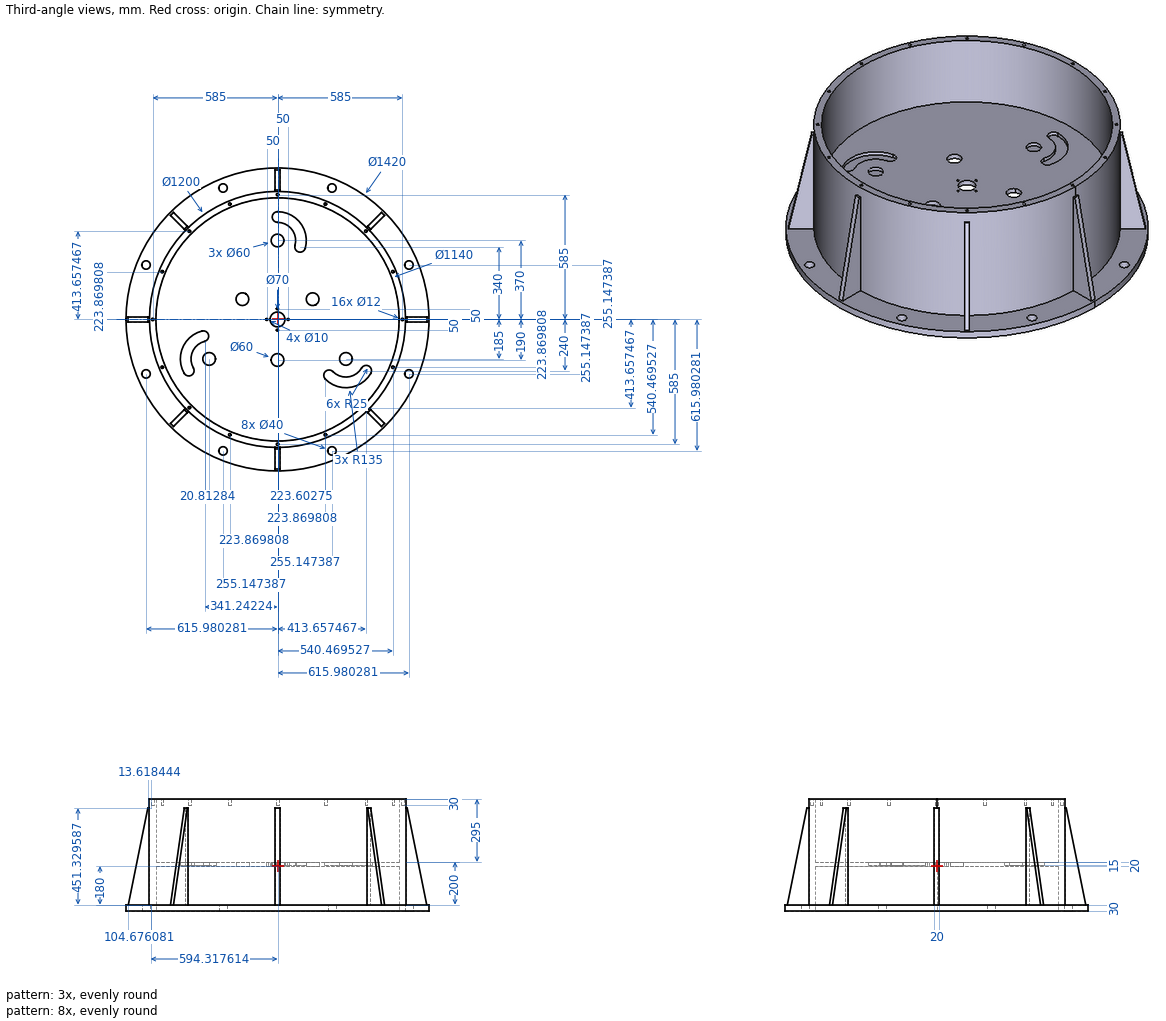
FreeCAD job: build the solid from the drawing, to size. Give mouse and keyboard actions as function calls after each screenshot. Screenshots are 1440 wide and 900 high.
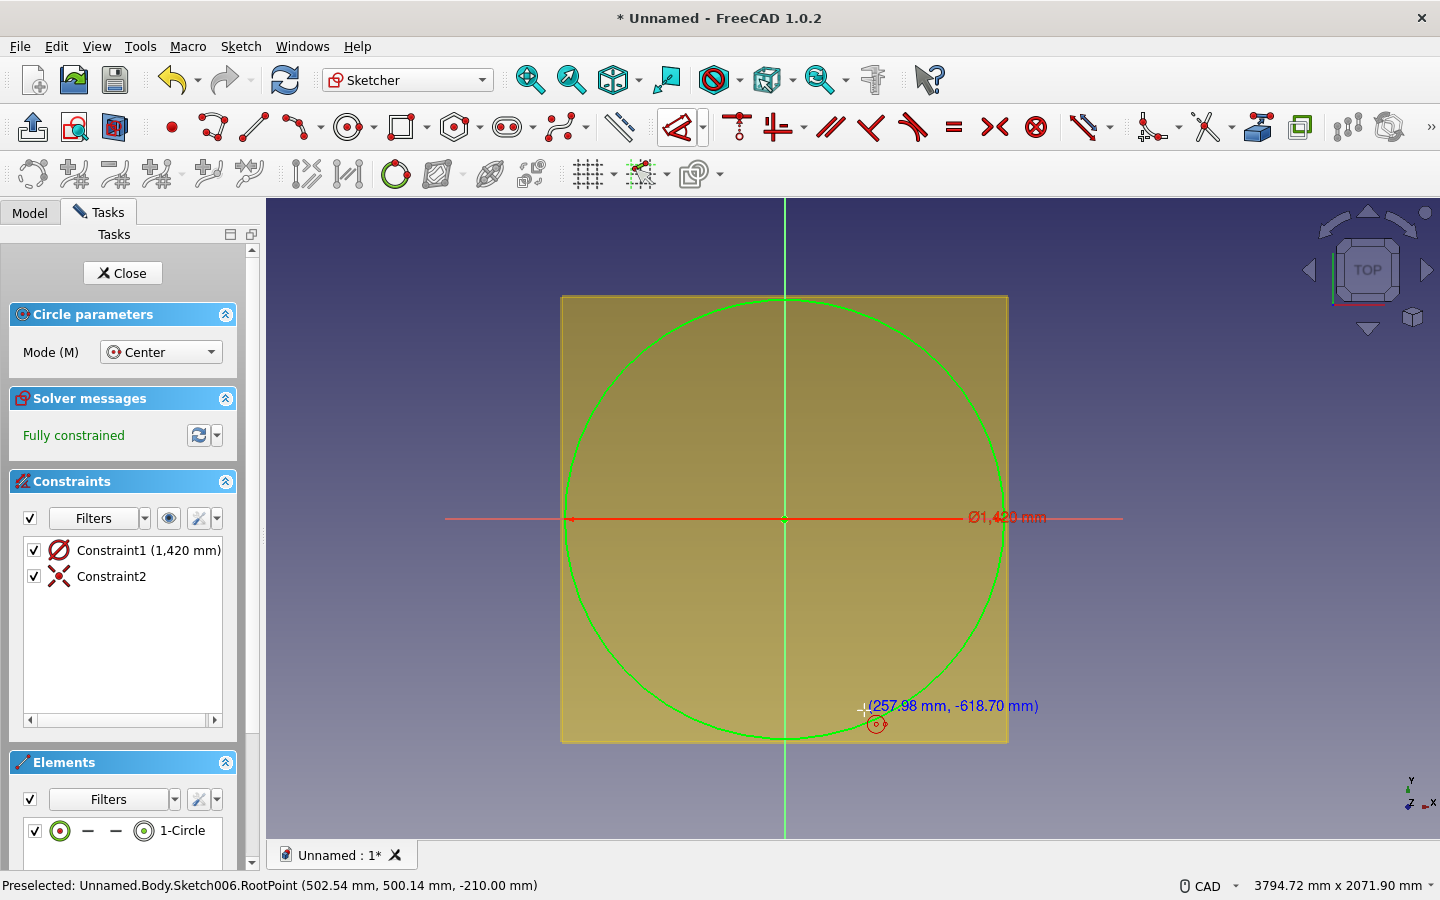
click(864, 710)
move(868, 706)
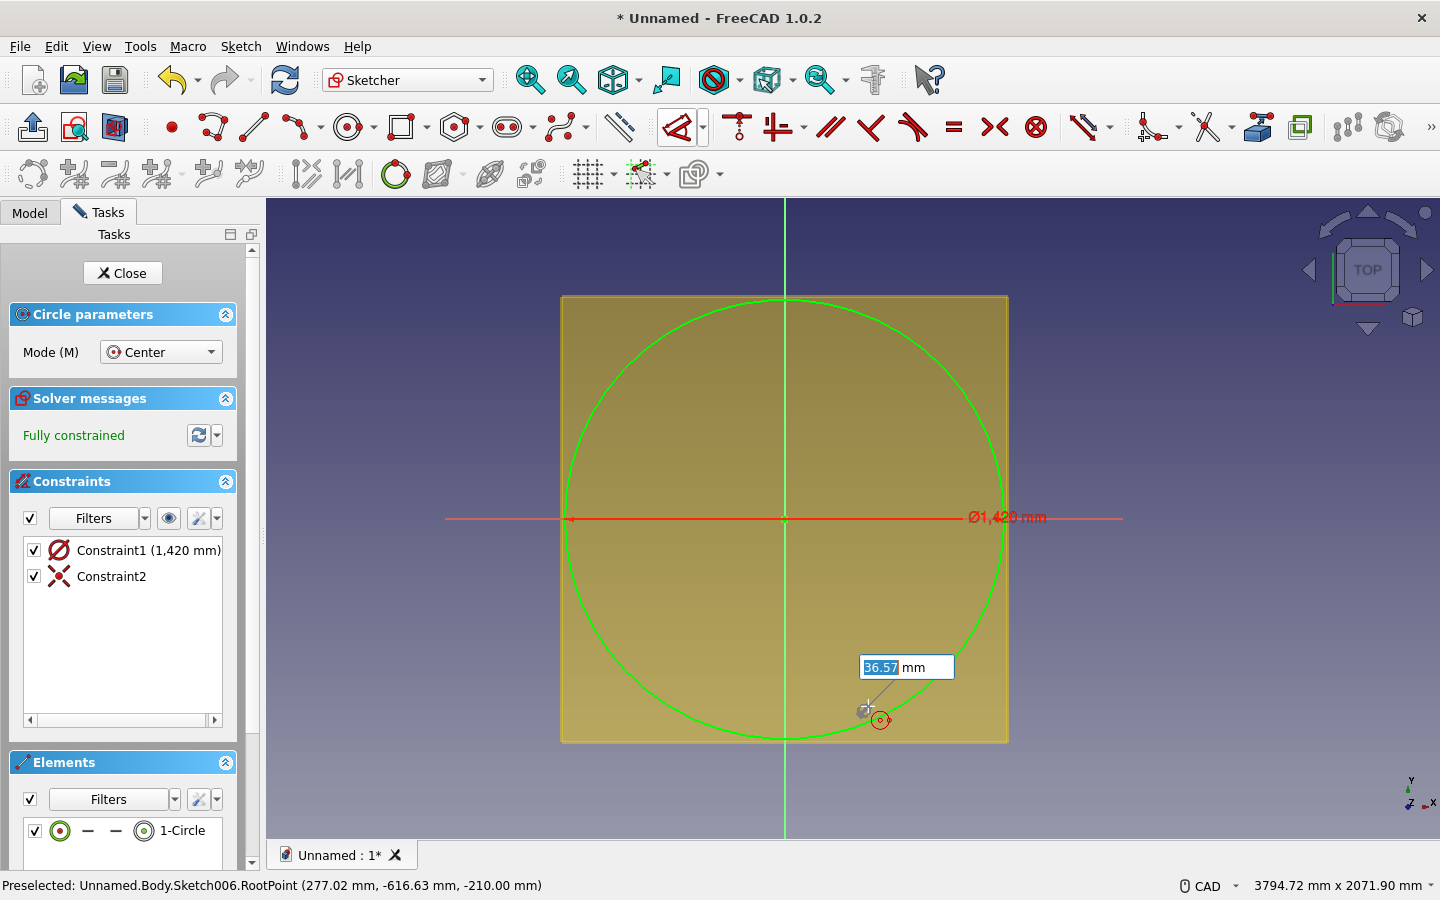
text(40)
key(Return)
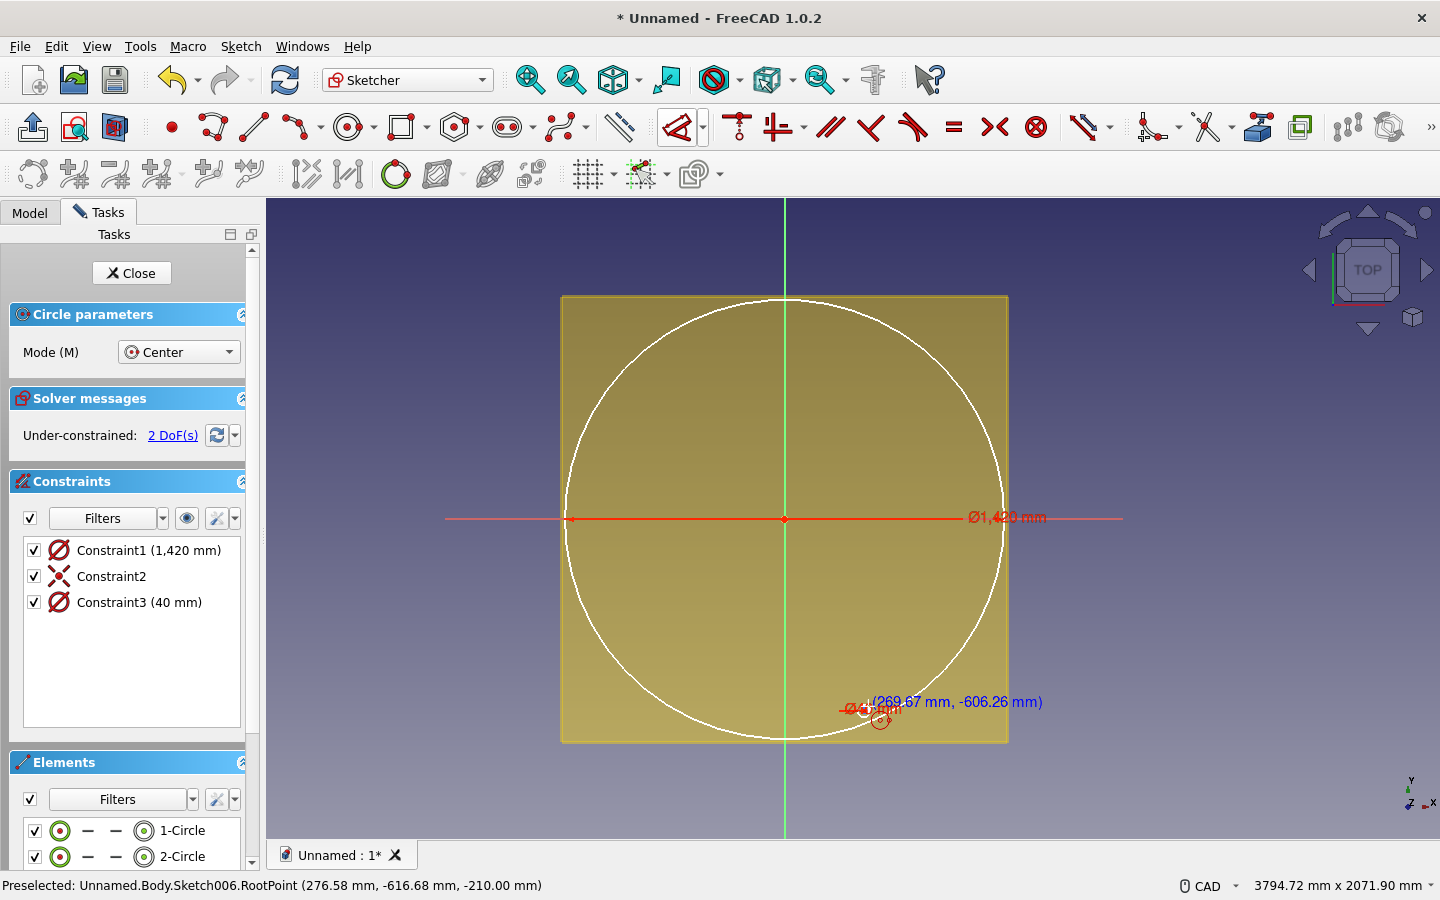
scroll(975, 598, up, 7)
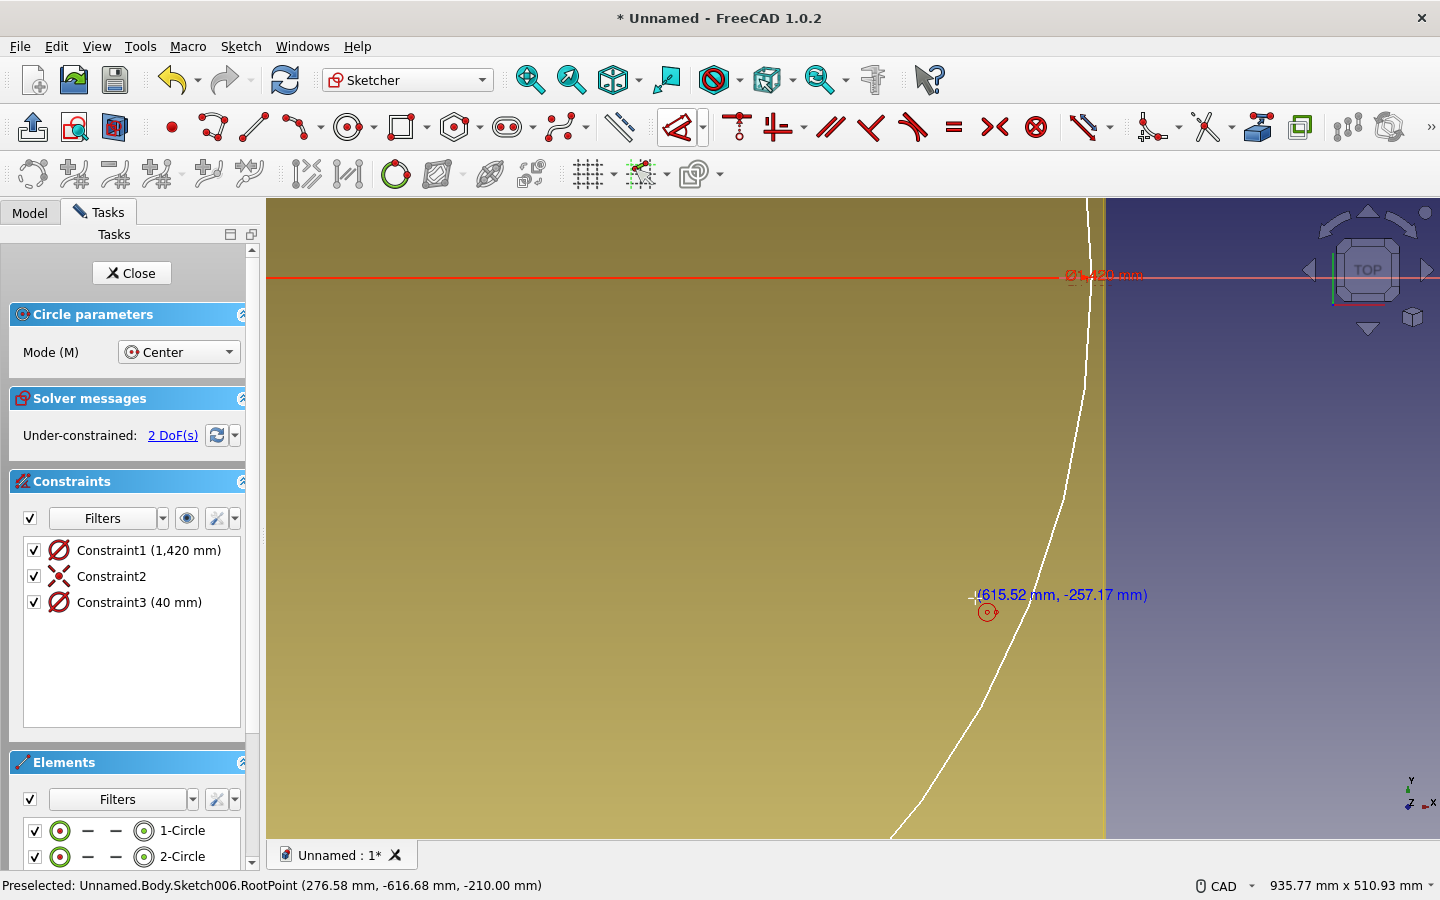
scroll(976, 597, down, 7)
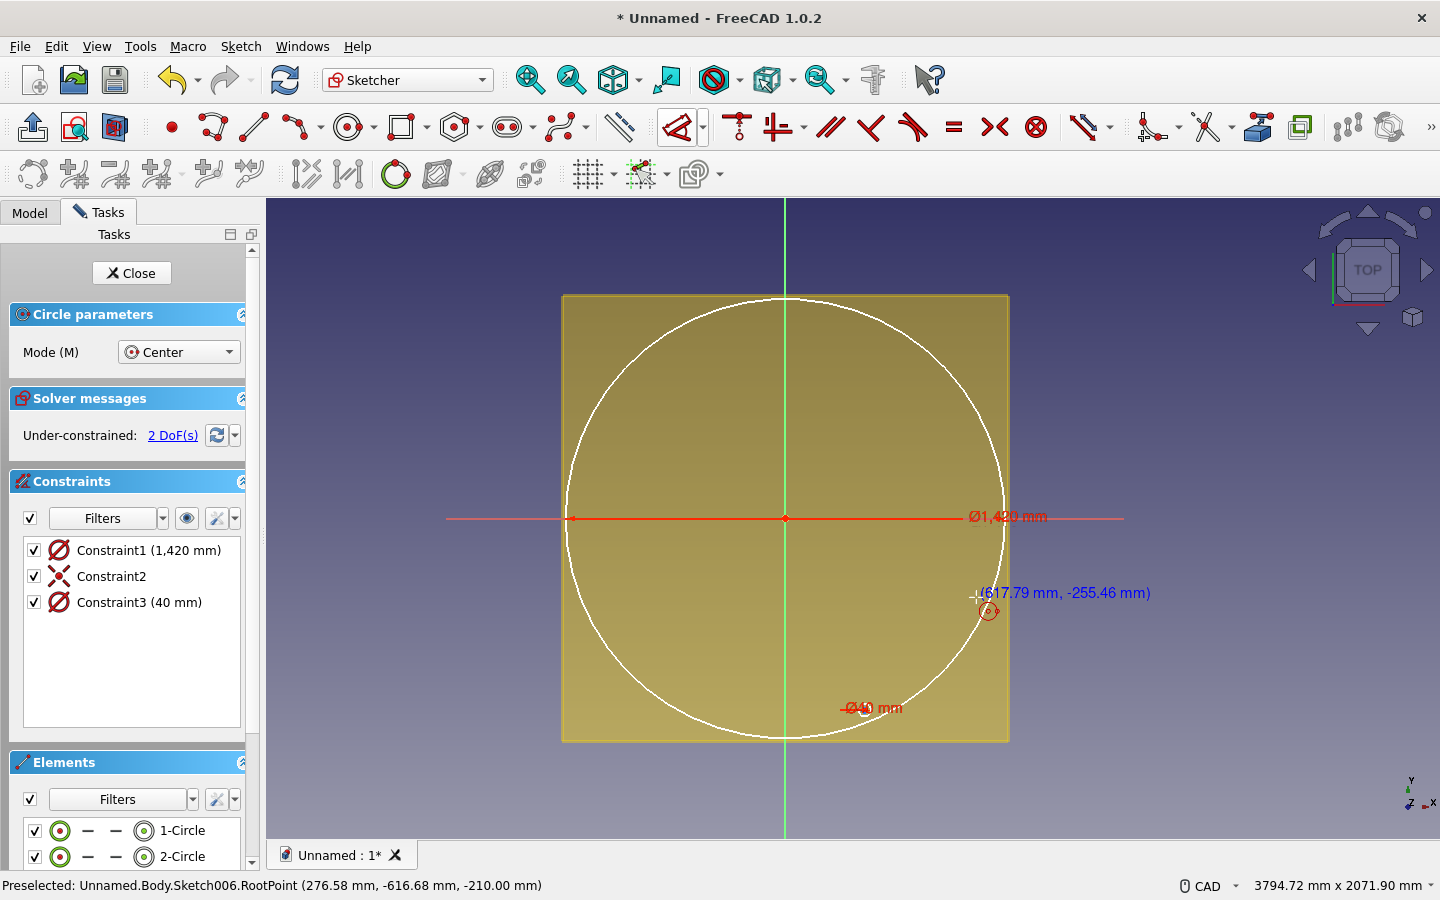
click(976, 598)
move(972, 593)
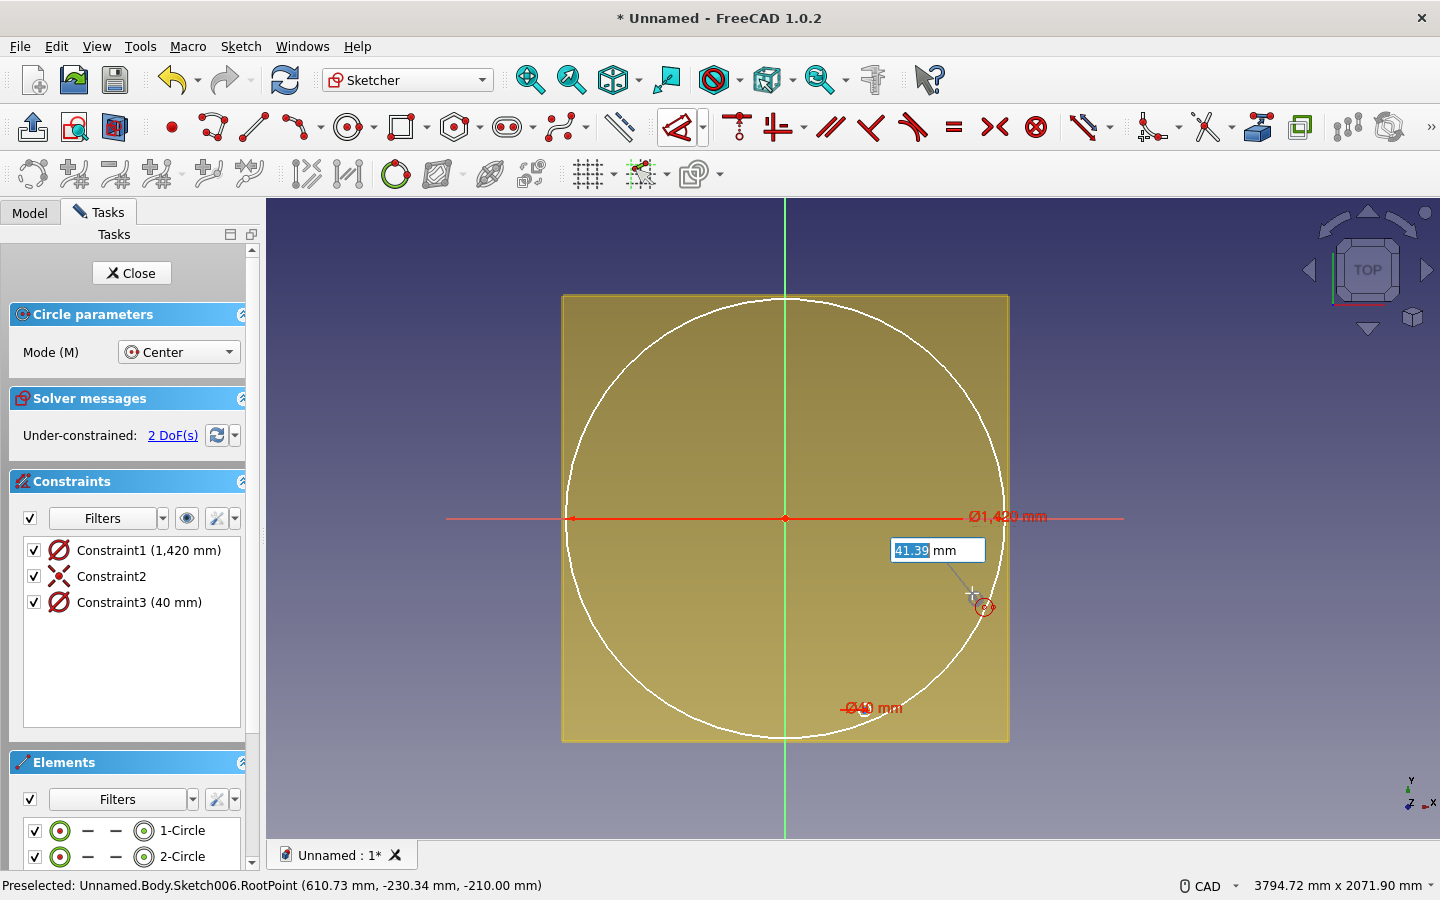
text(40)
key(Return)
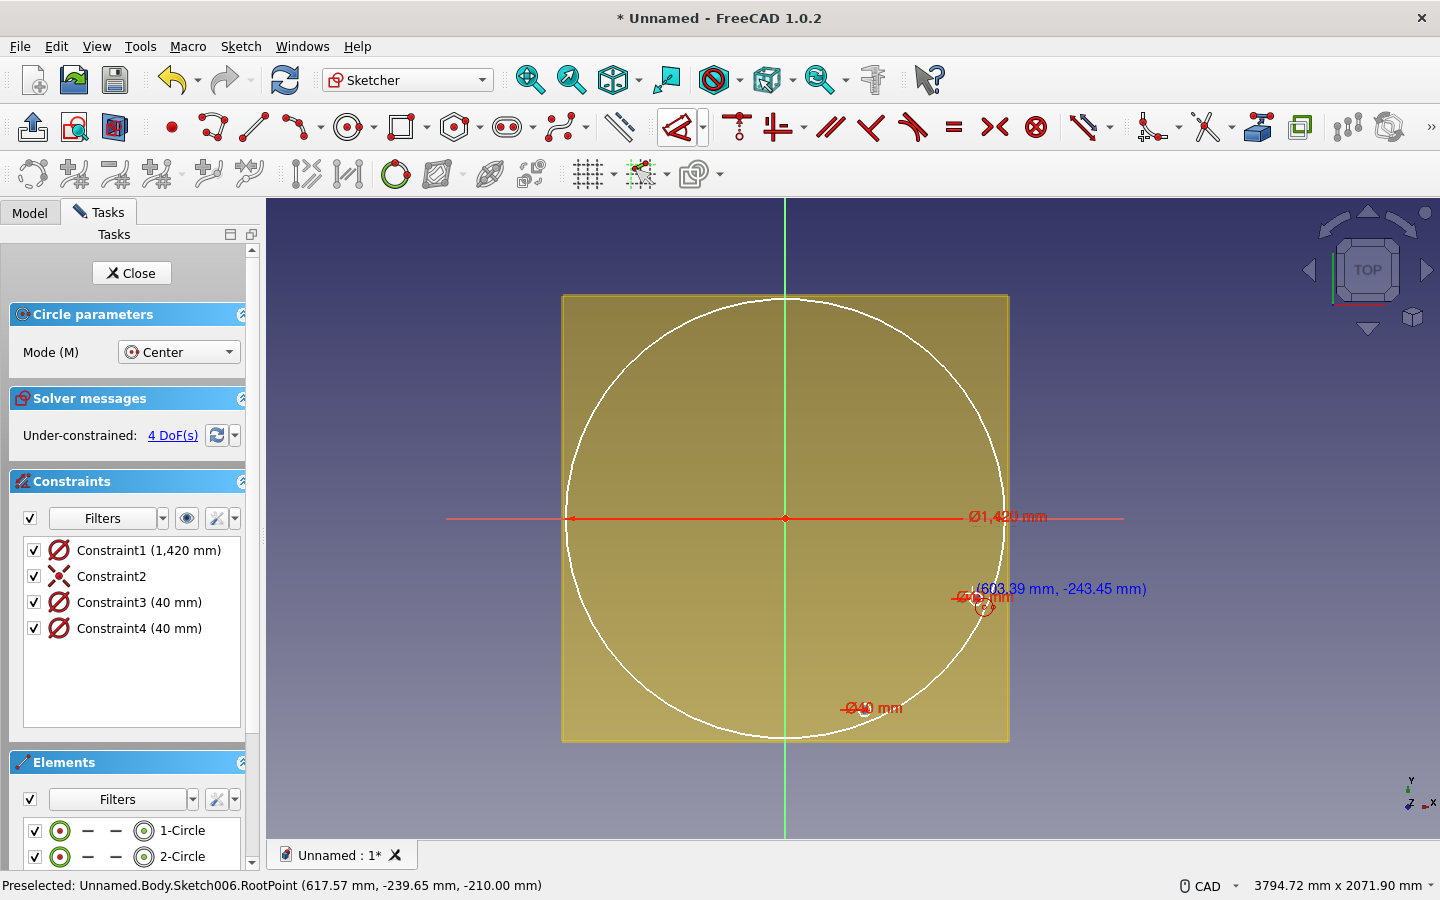
scroll(706, 709, up, 7)